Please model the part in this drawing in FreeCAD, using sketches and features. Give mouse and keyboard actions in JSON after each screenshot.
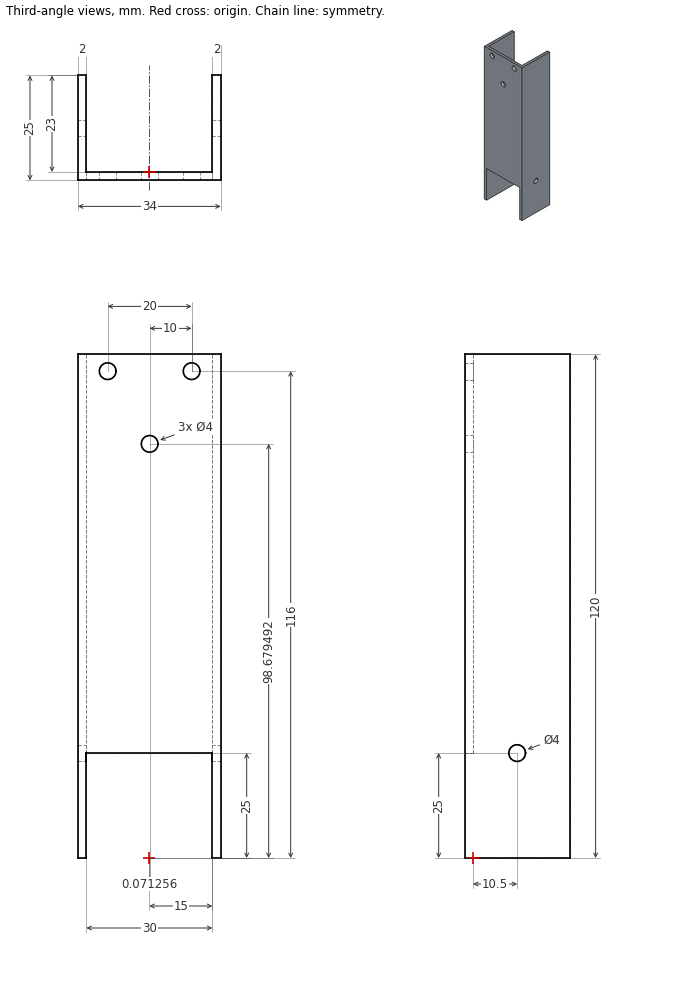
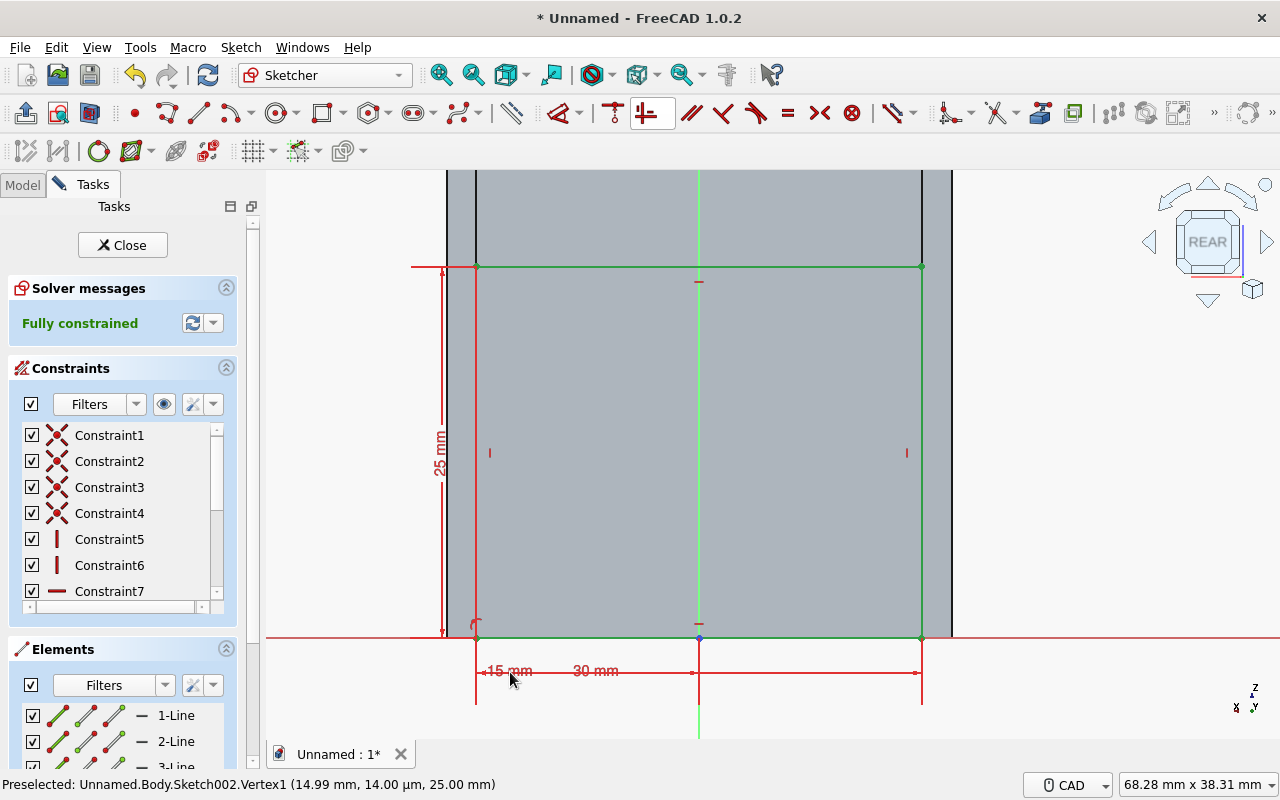
{"action": "left_click", "coordinate": [123, 245]}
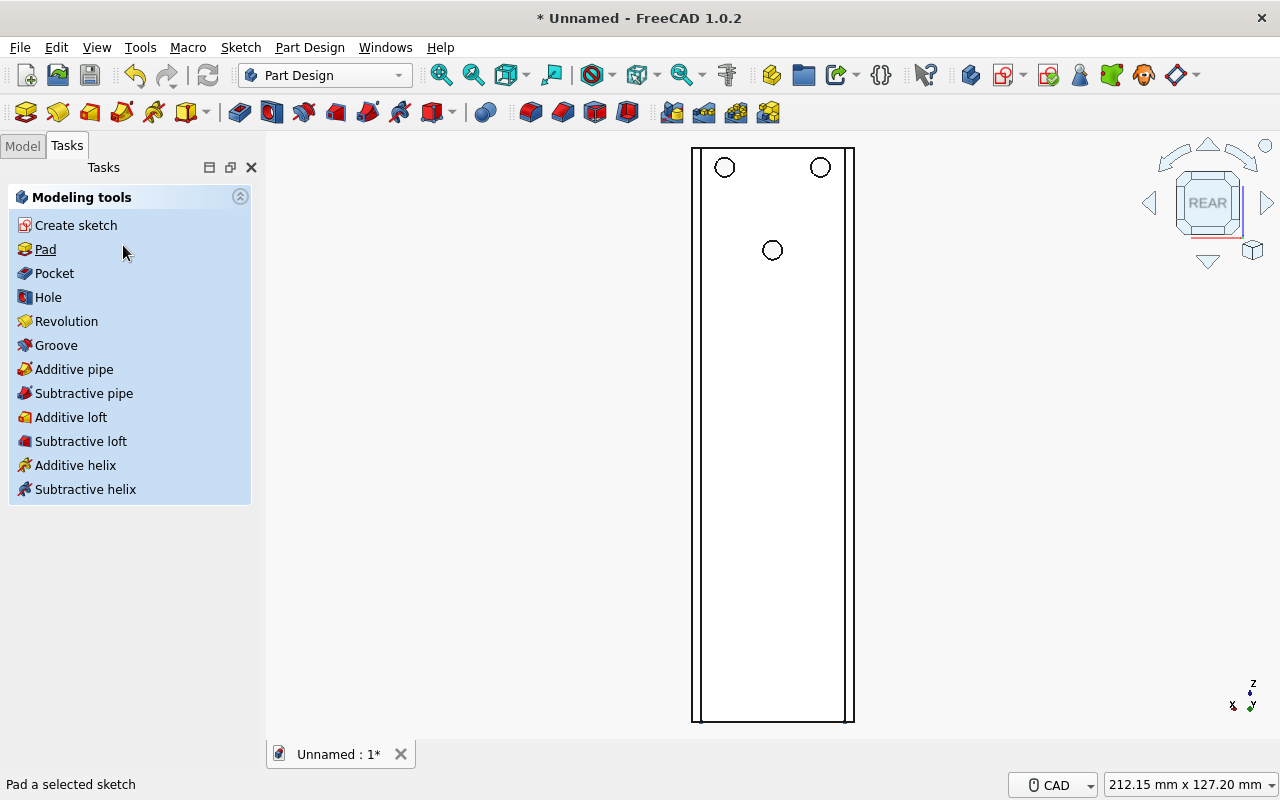
{"action": "left_click", "coordinate": [240, 112]}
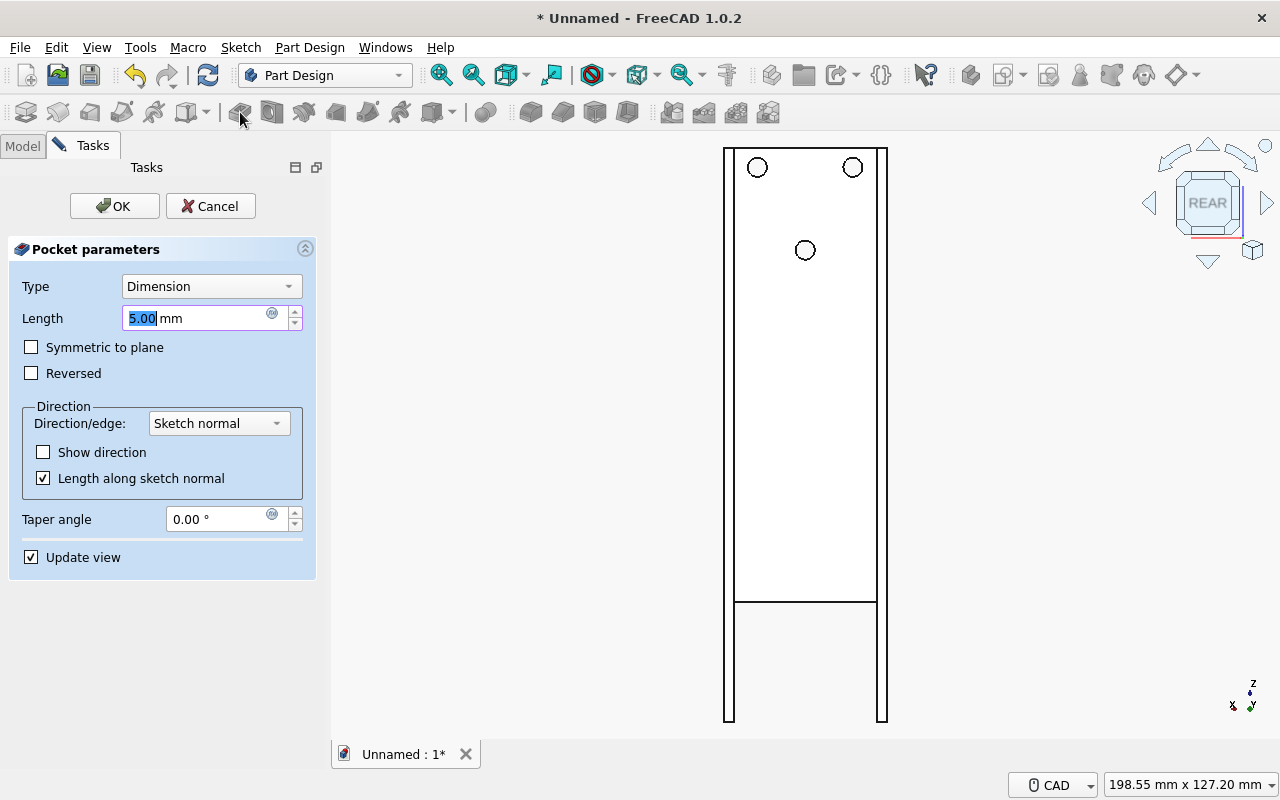
{"action": "left_click", "coordinate": [212, 286]}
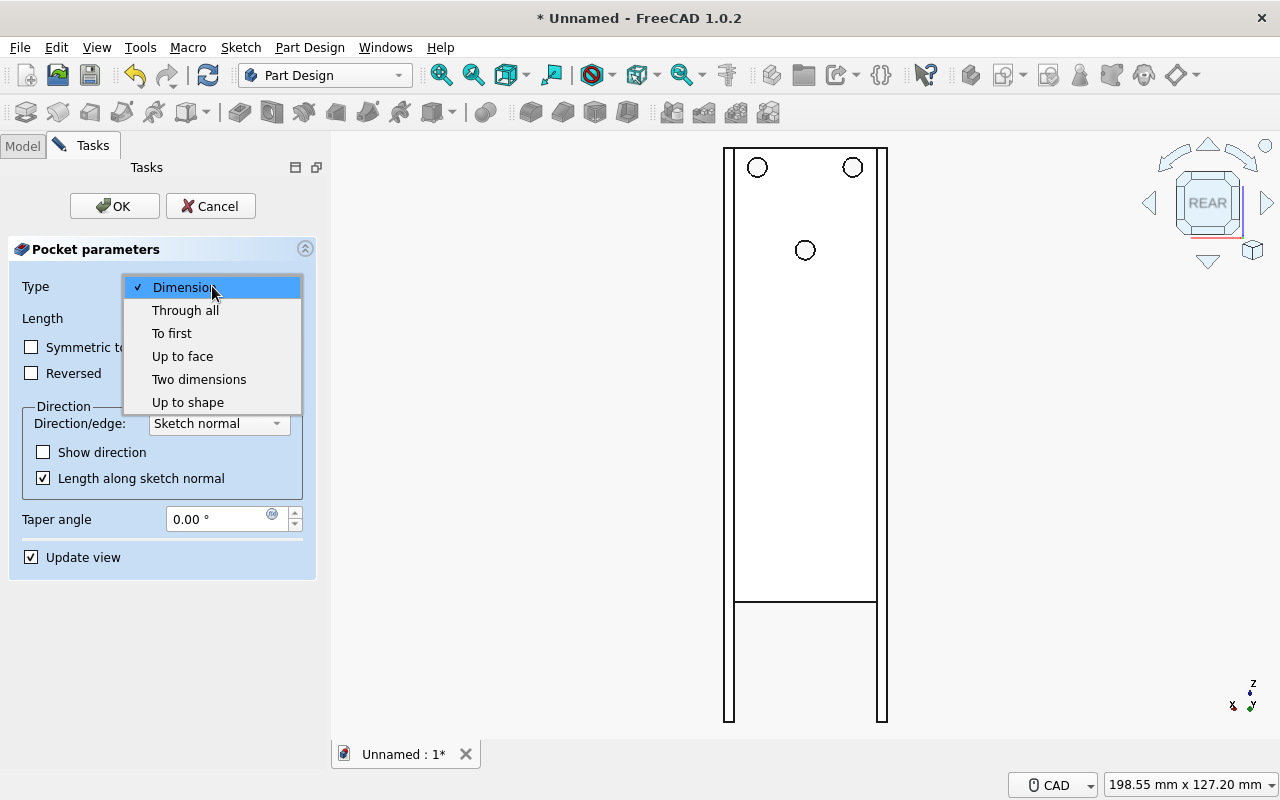
{"action": "left_click", "coordinate": [212, 310]}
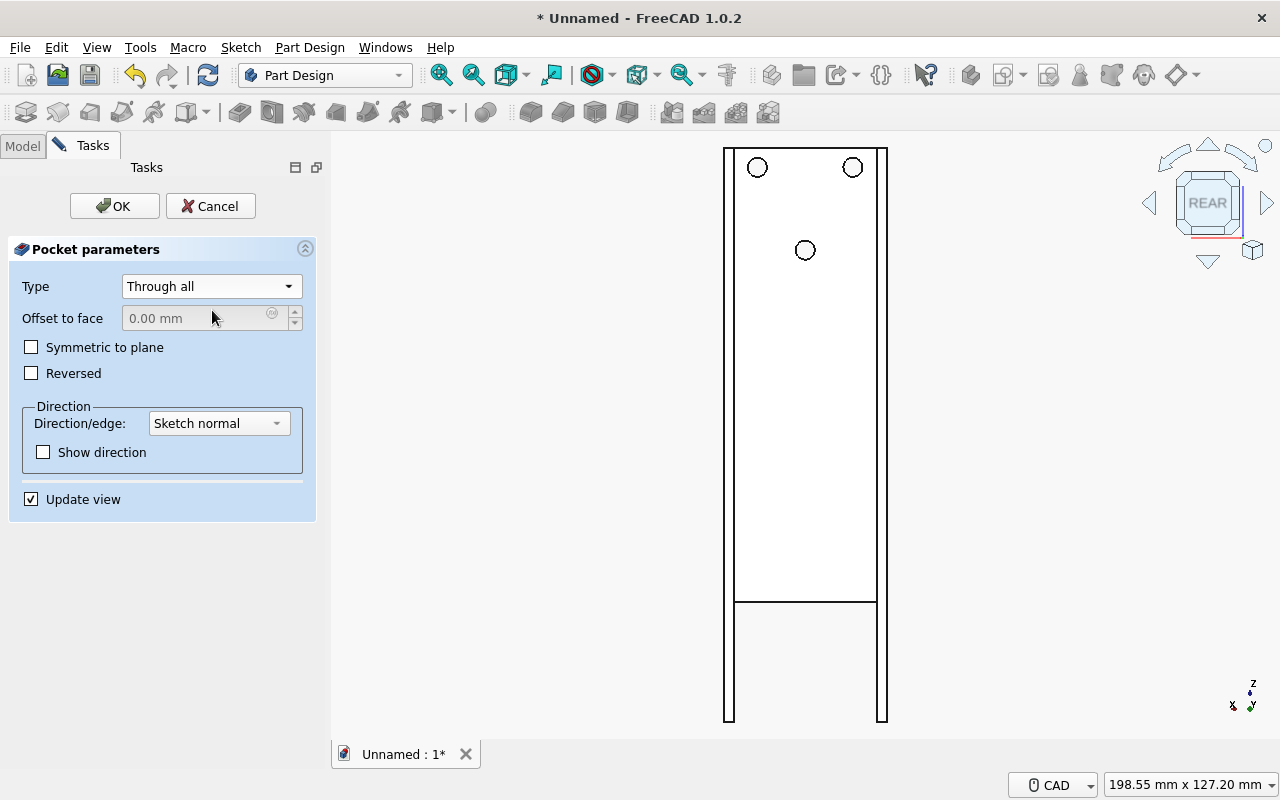
{"action": "left_click", "coordinate": [115, 206]}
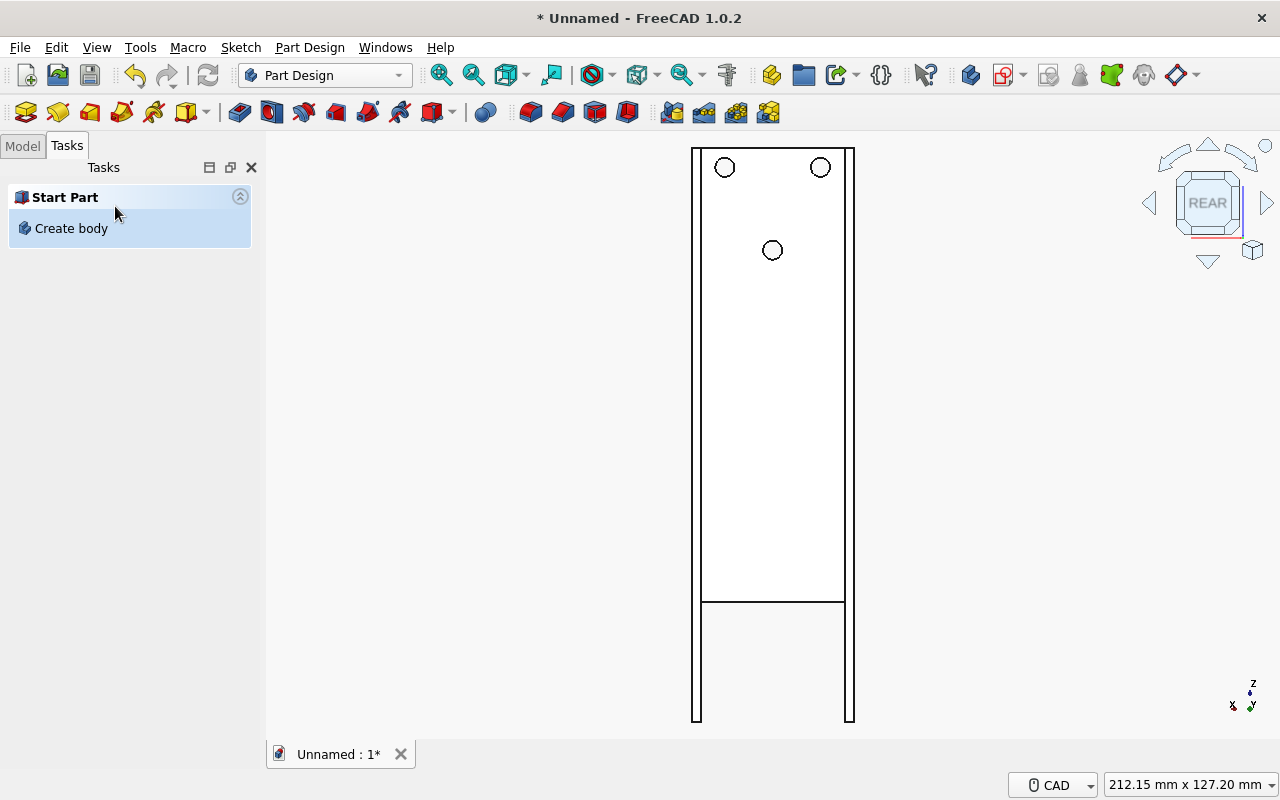
{"action": "key", "text": "0"}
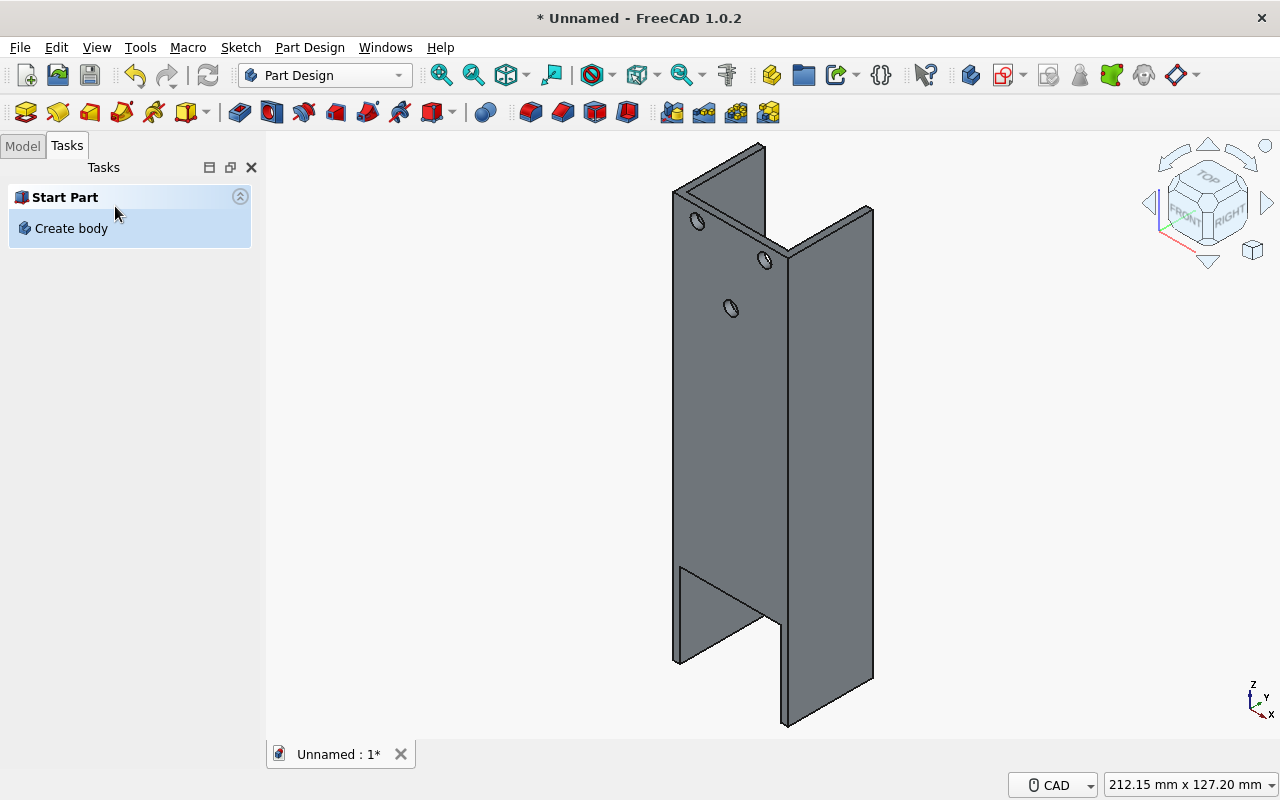
{"action": "left_click", "coordinate": [830, 333]}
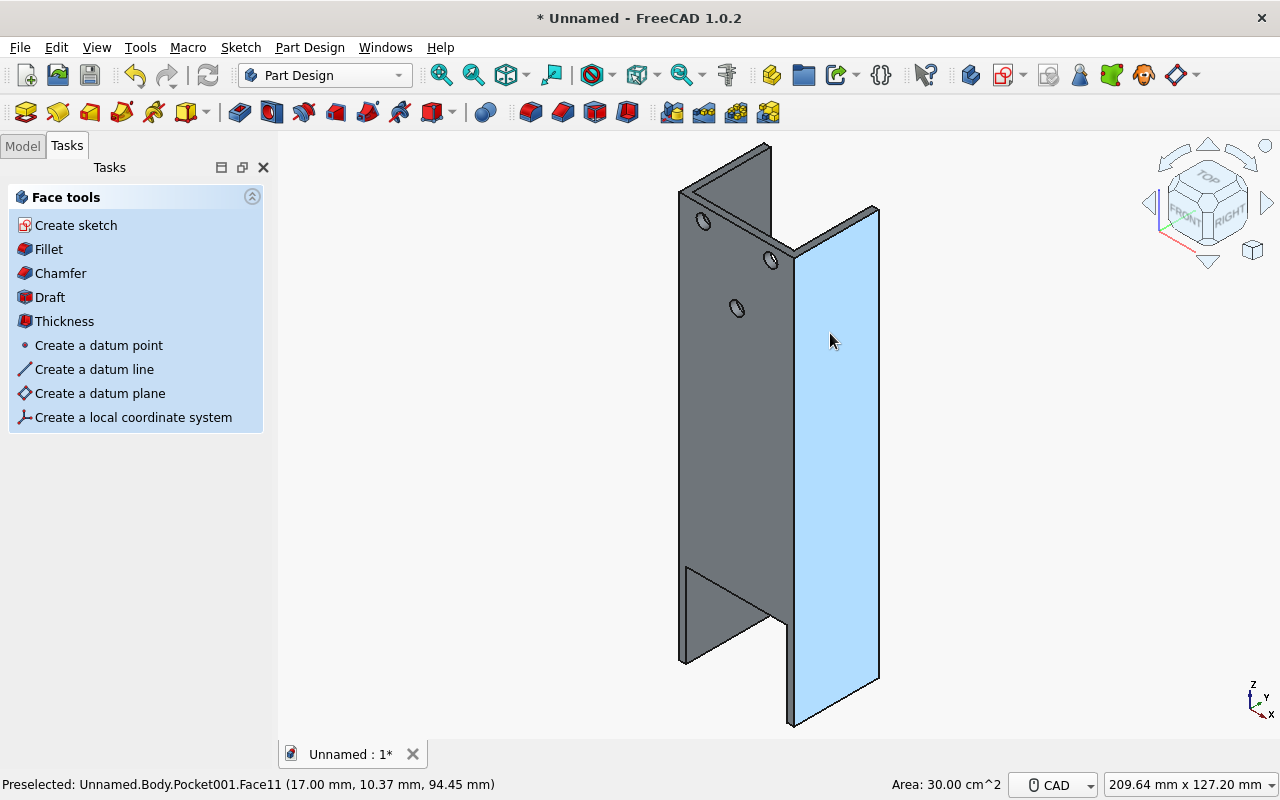
{"action": "left_click", "coordinate": [1004, 76]}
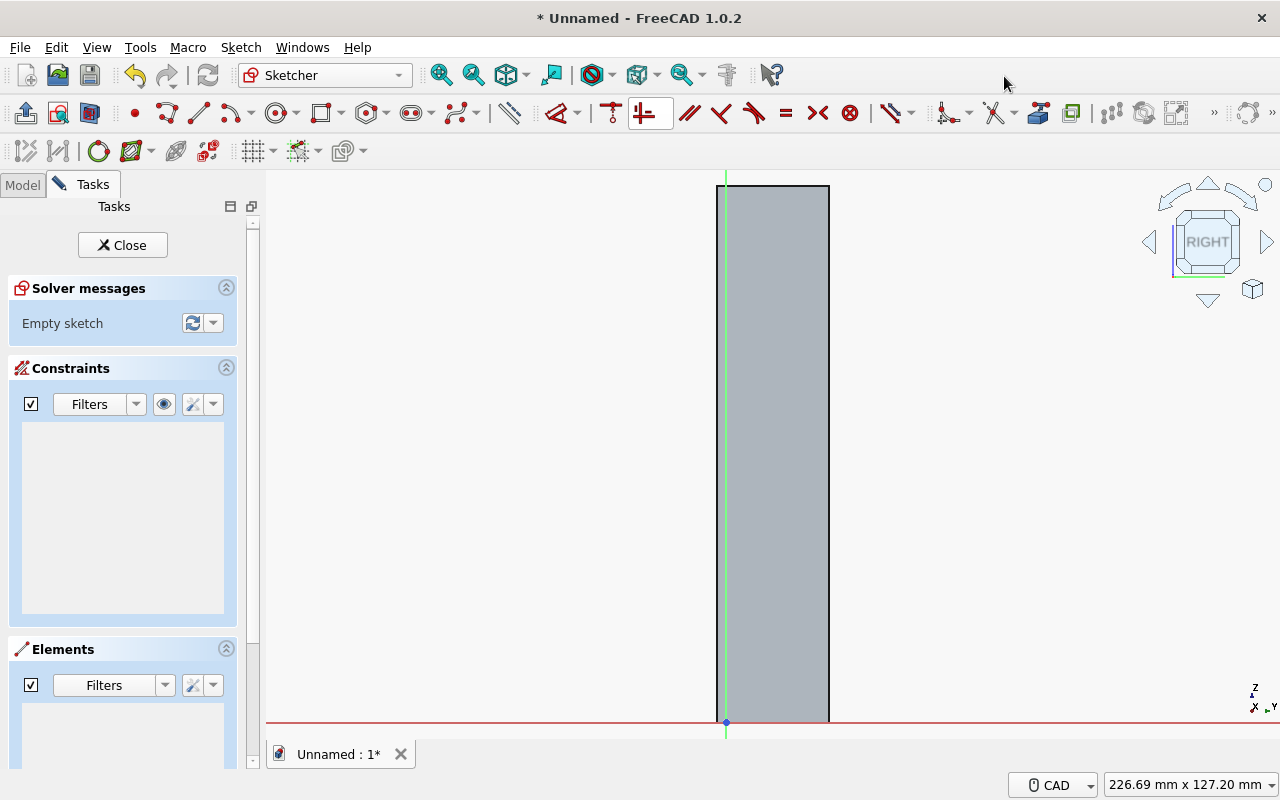
{"action": "scroll", "coordinate": [777, 619], "scroll_direction": "up", "scroll_amount": 15}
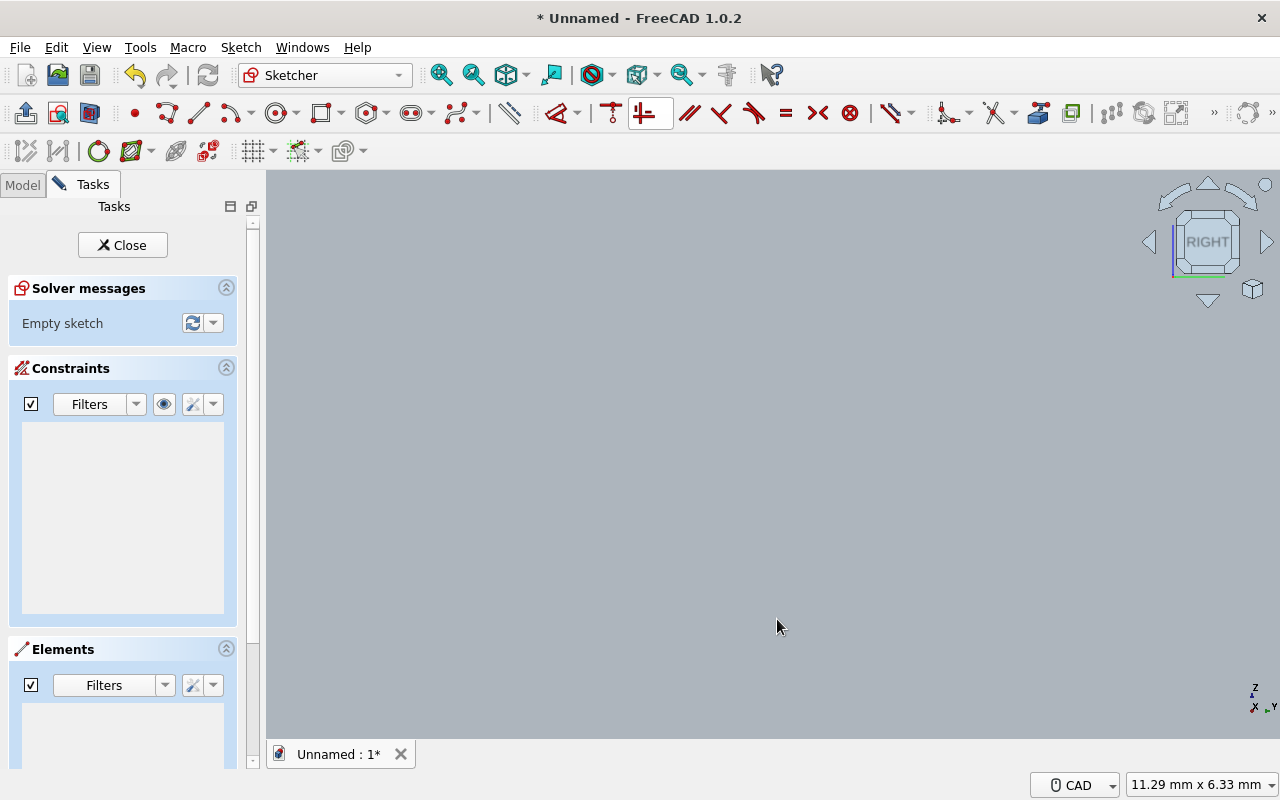
{"action": "left_click", "coordinate": [276, 114]}